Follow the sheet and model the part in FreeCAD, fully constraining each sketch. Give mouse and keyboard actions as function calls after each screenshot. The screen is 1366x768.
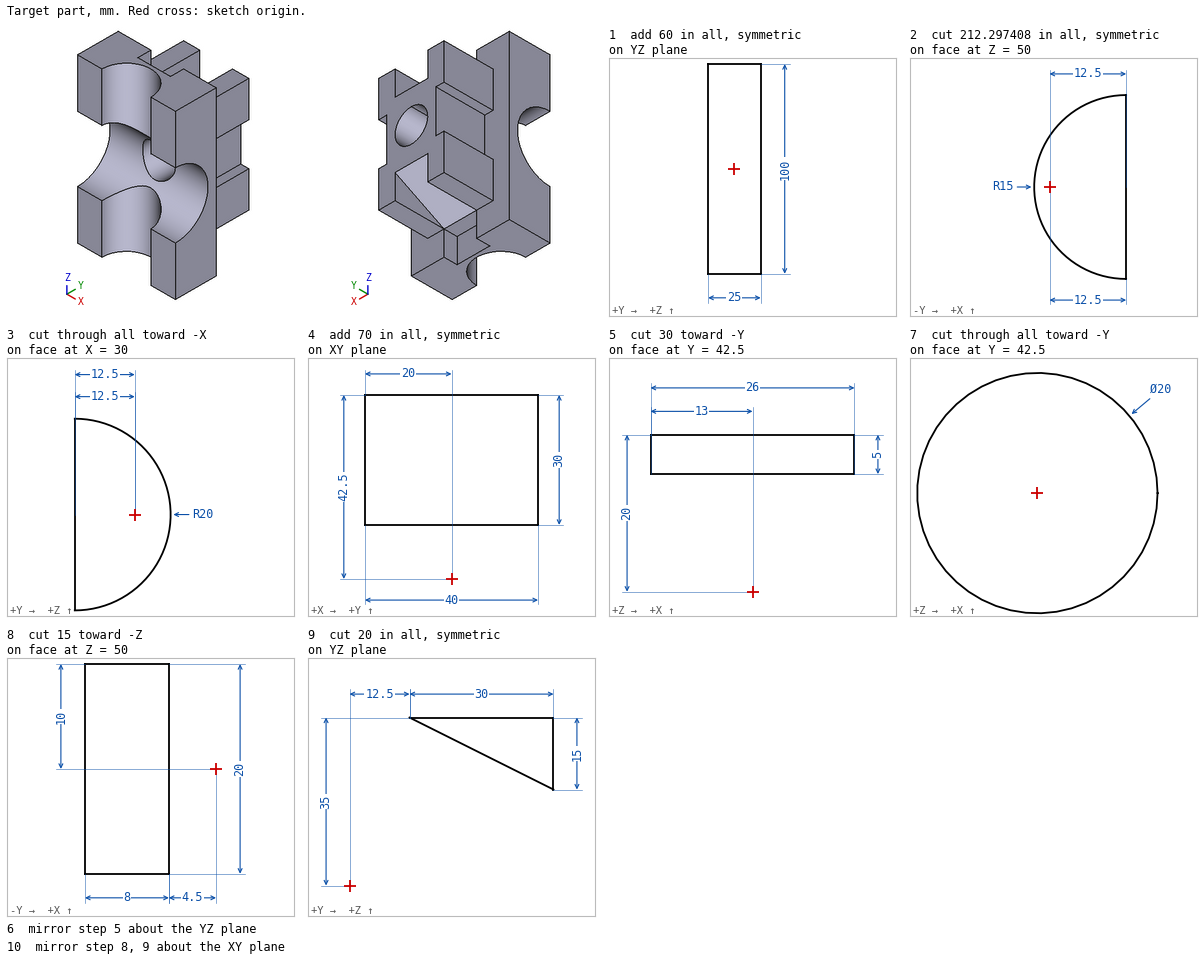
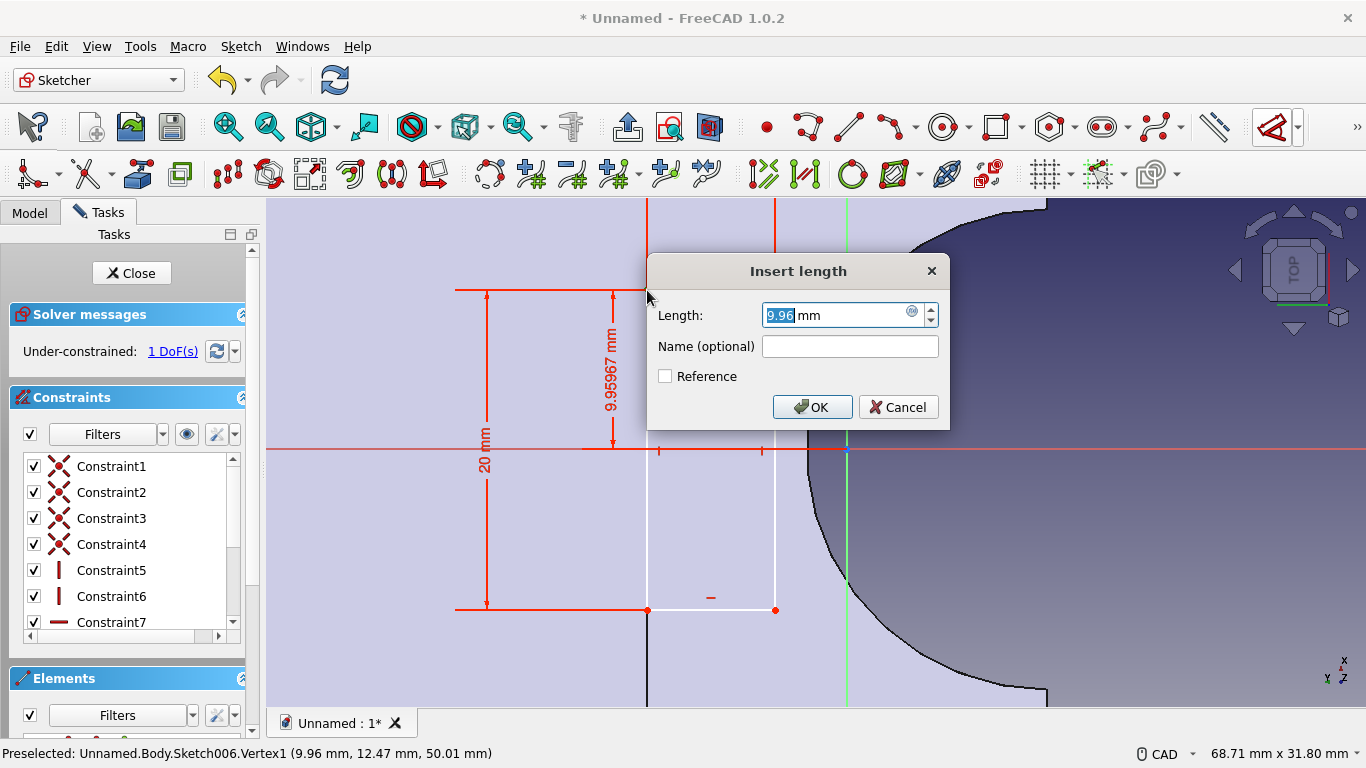
text(10)
key(Return)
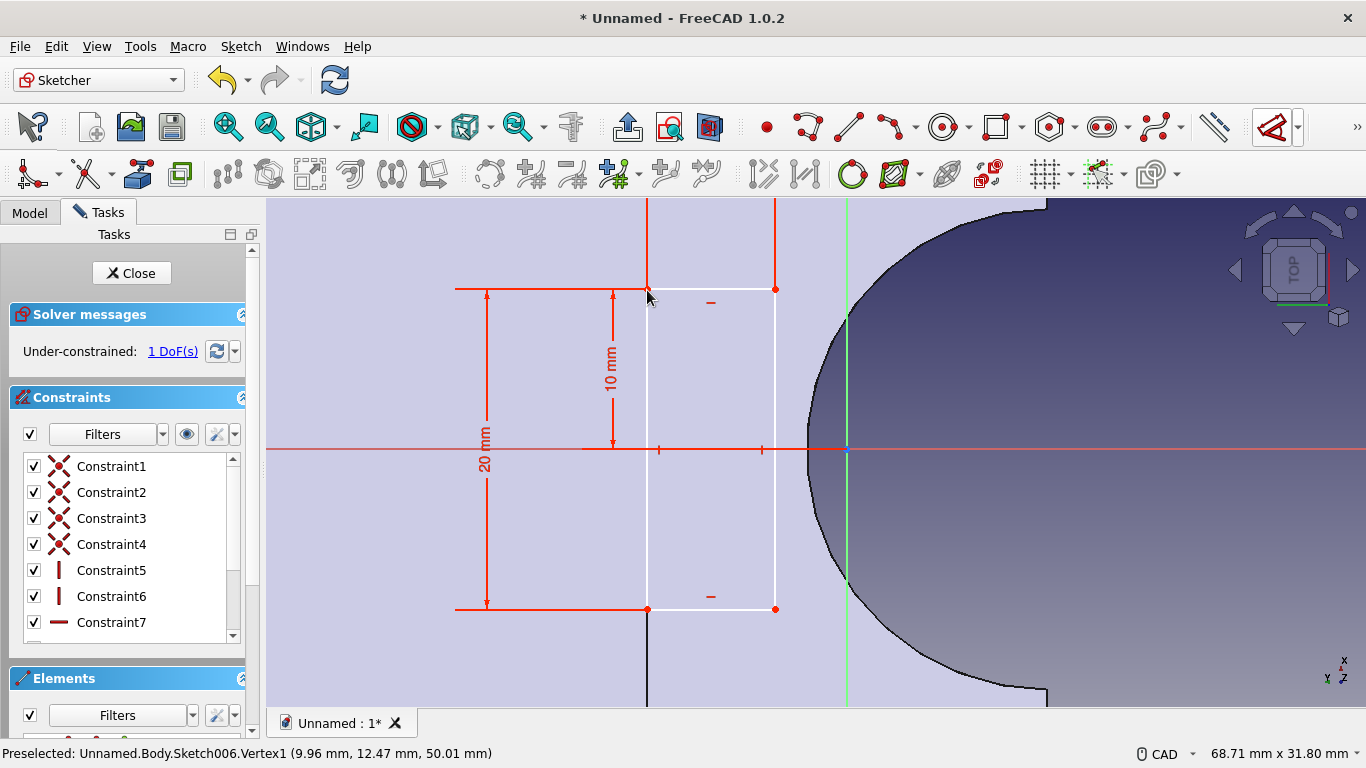
click(775, 610)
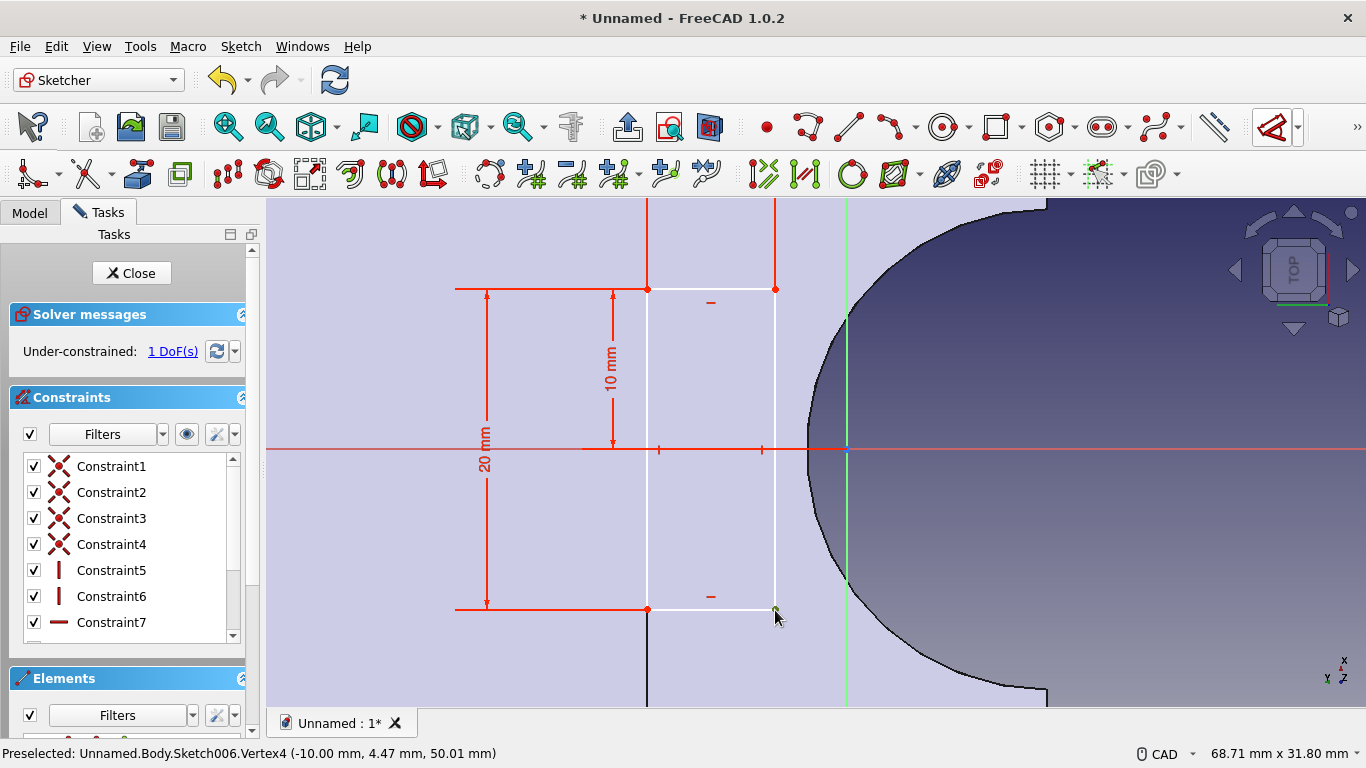
key(l)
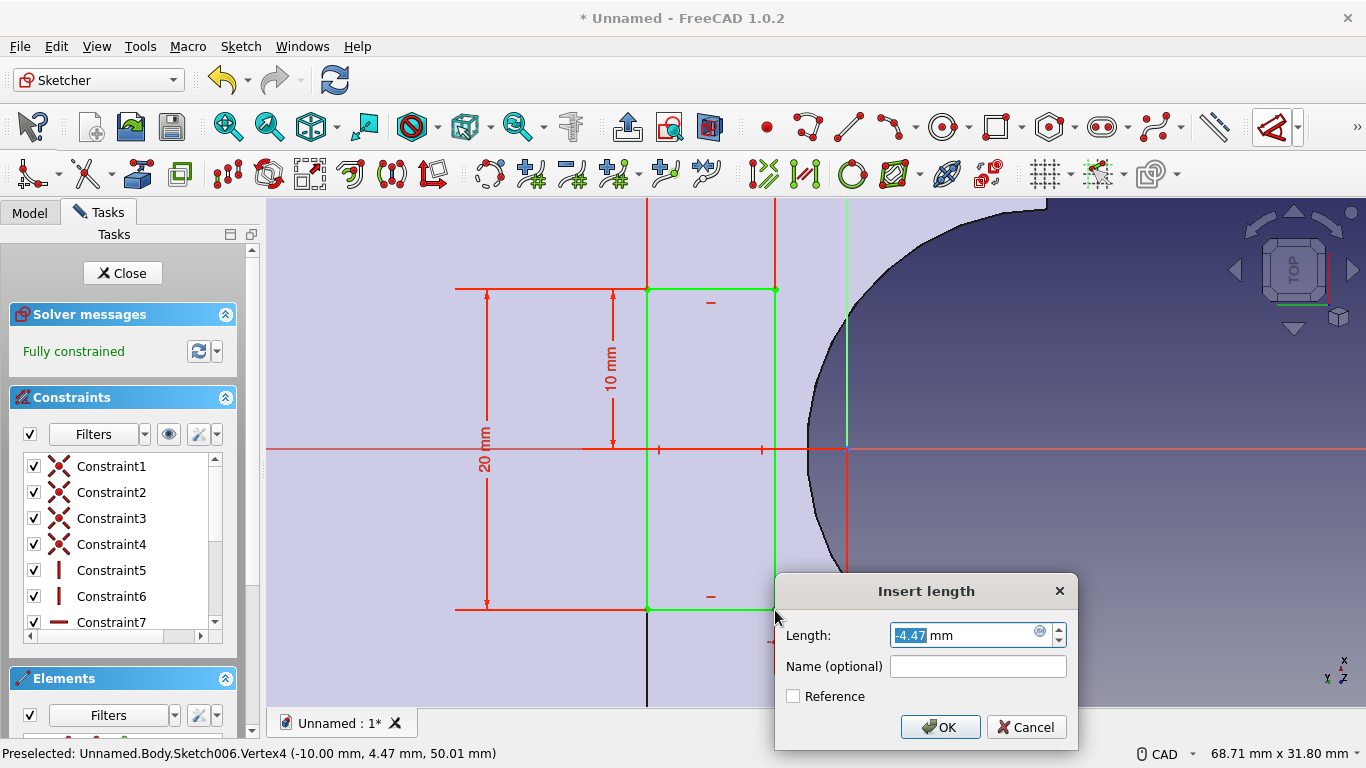
text(-4.5)
key(Return)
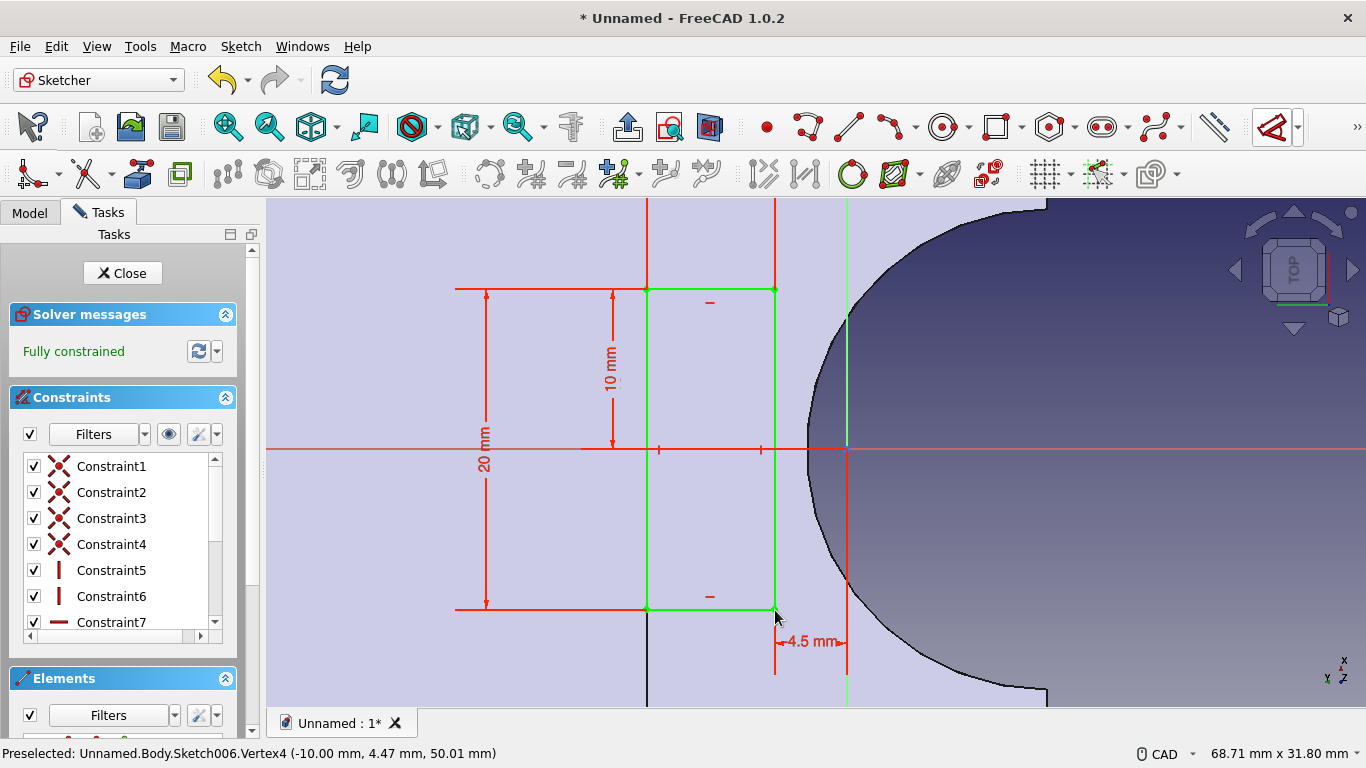
click(123, 273)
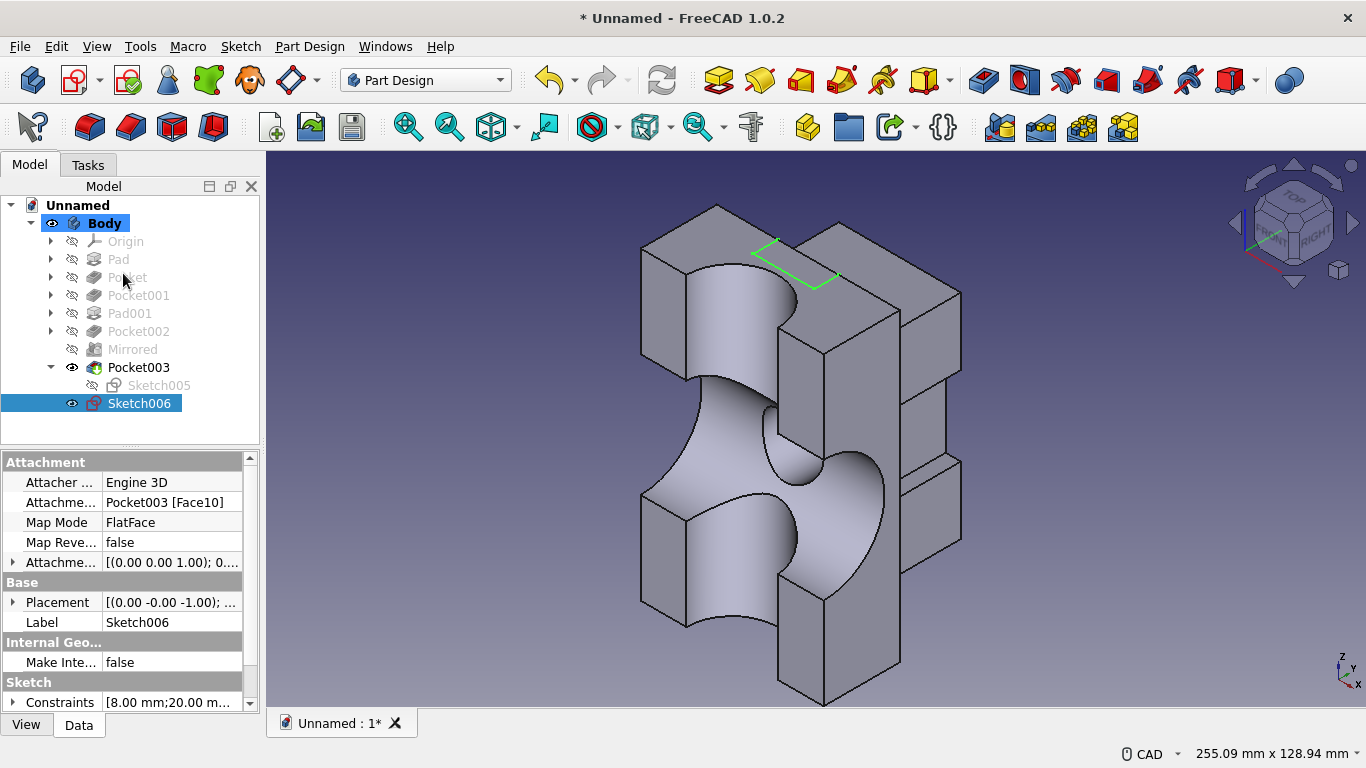
click(984, 80)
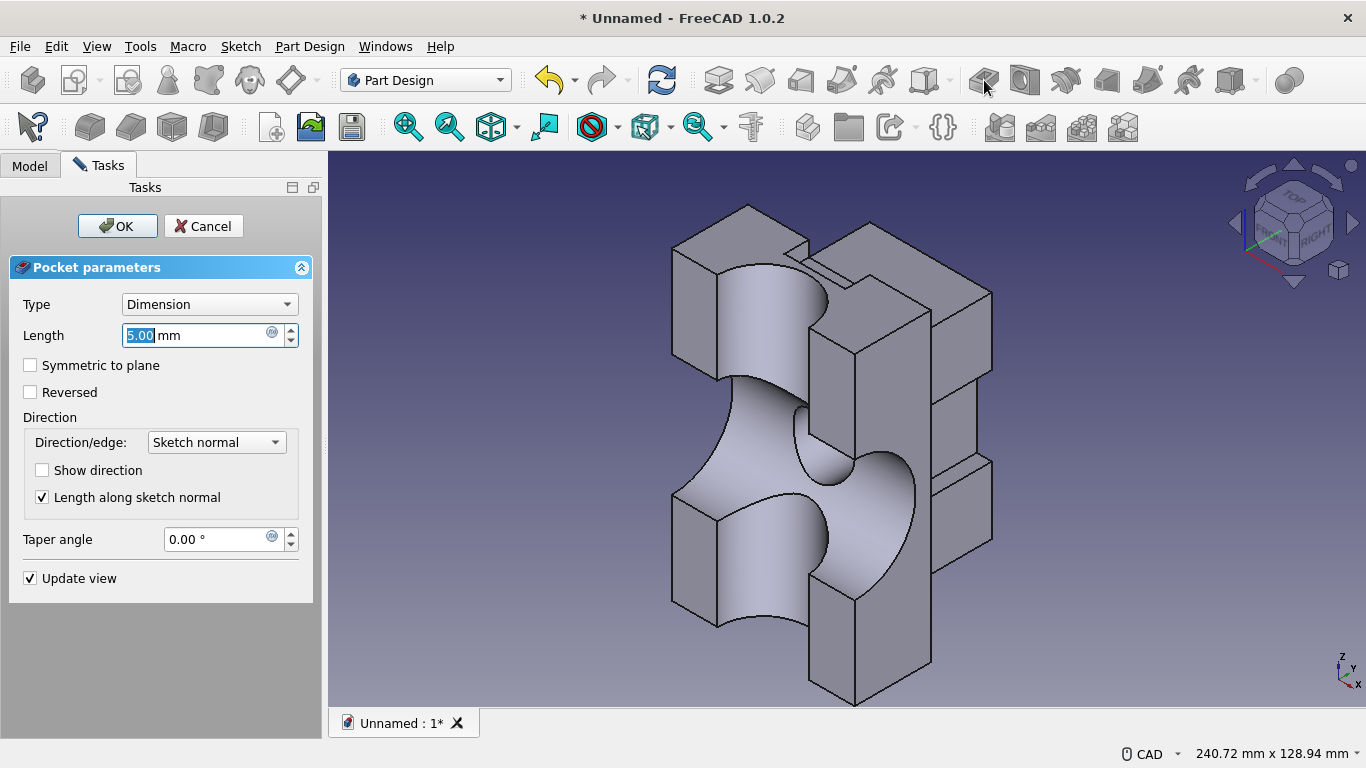
text(15)
key(Tab)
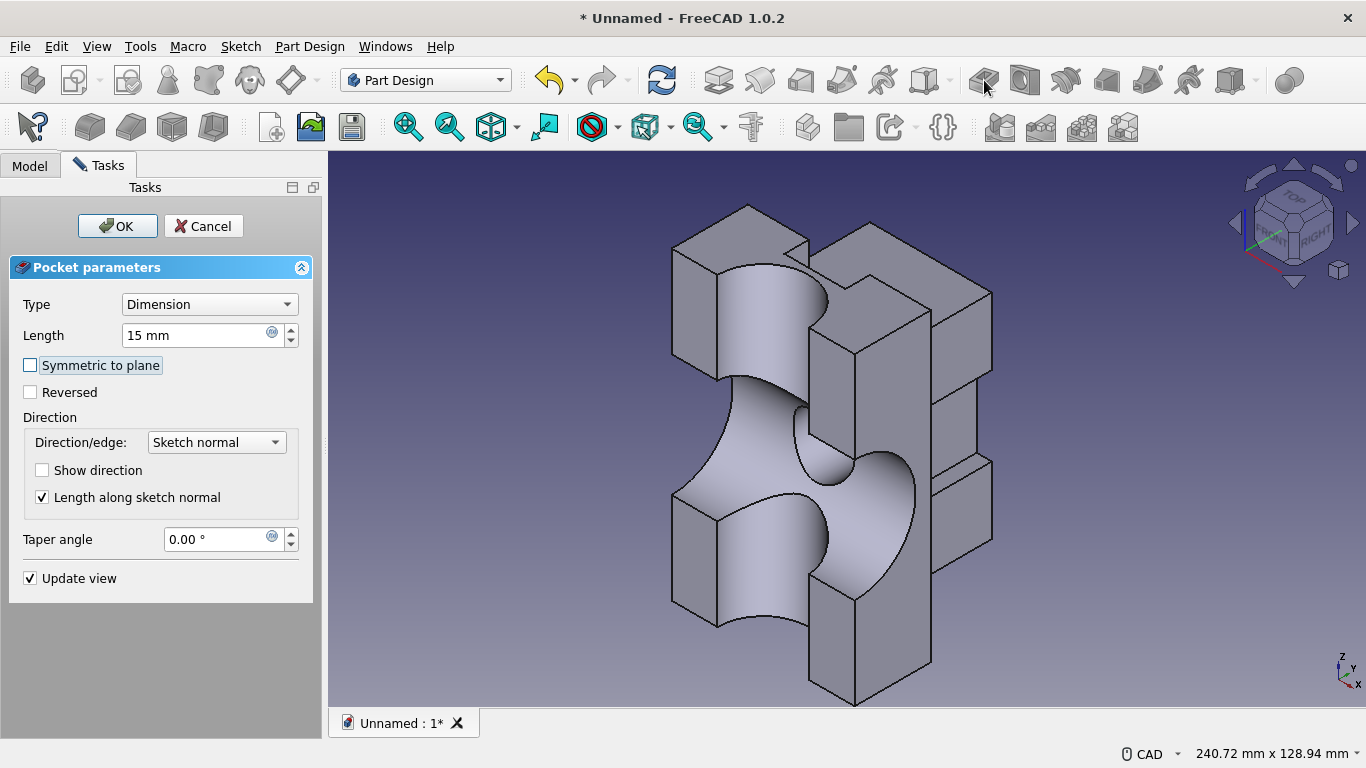
click(118, 226)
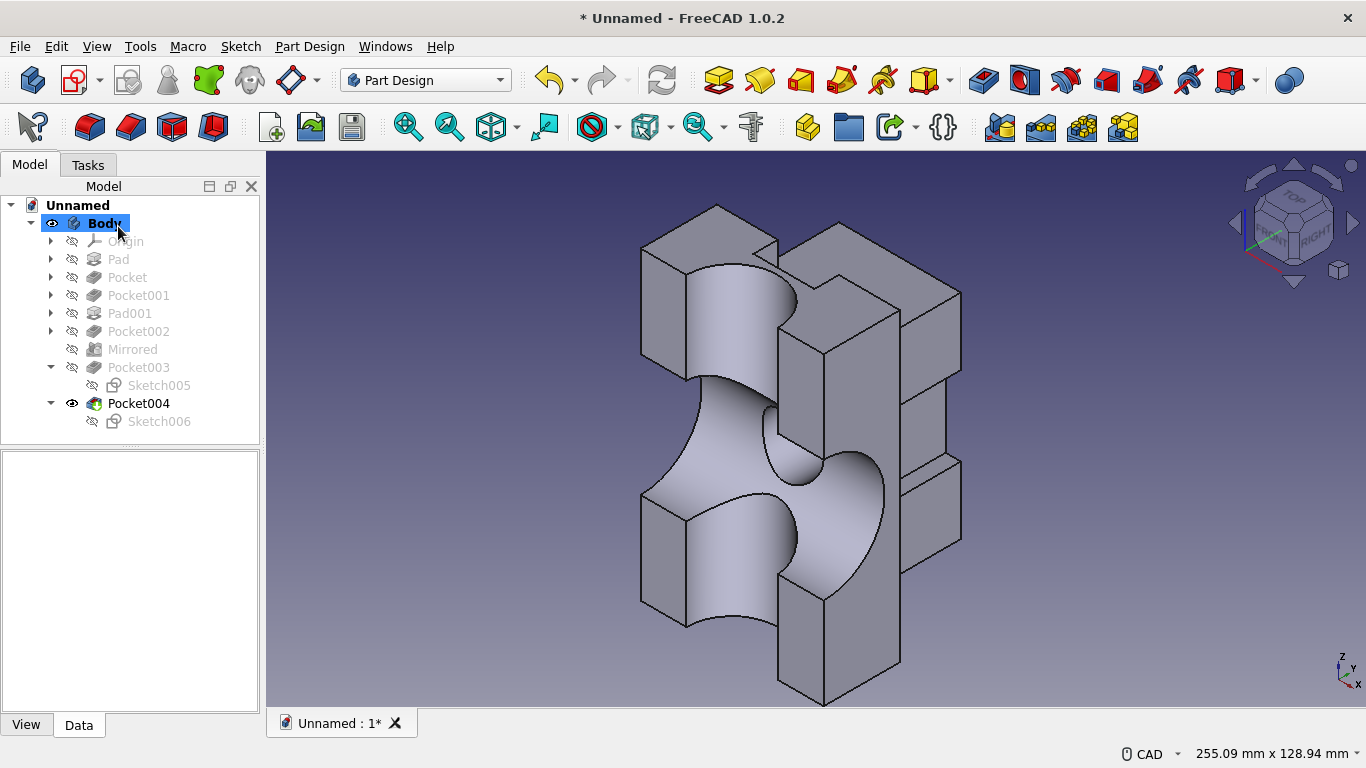
click(74, 80)